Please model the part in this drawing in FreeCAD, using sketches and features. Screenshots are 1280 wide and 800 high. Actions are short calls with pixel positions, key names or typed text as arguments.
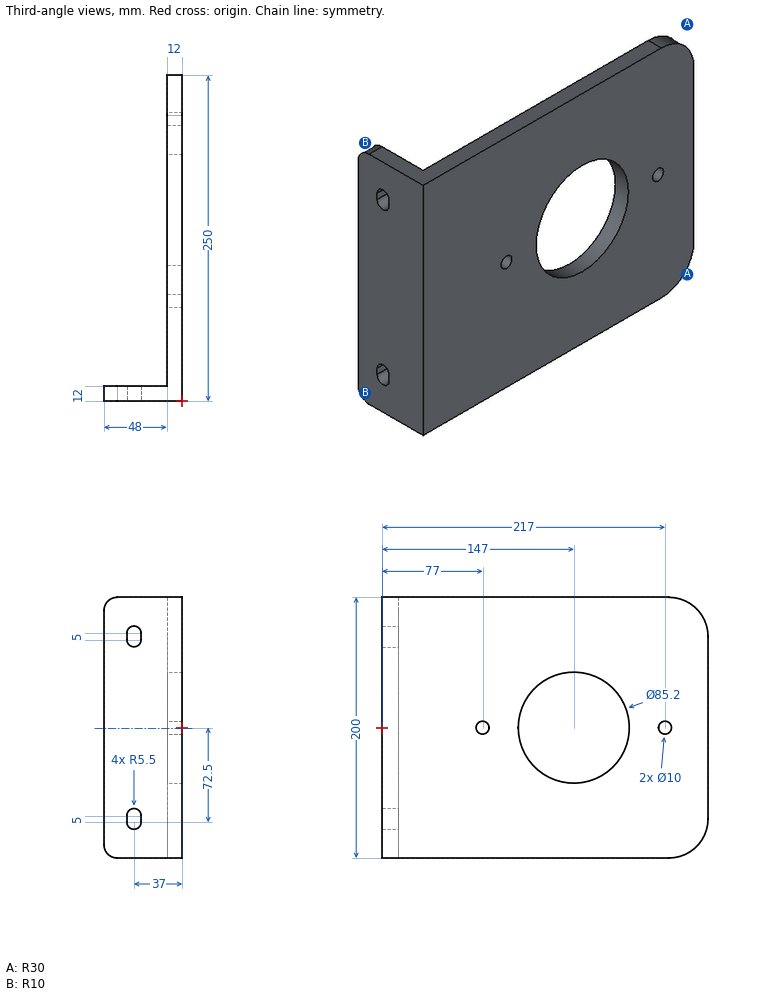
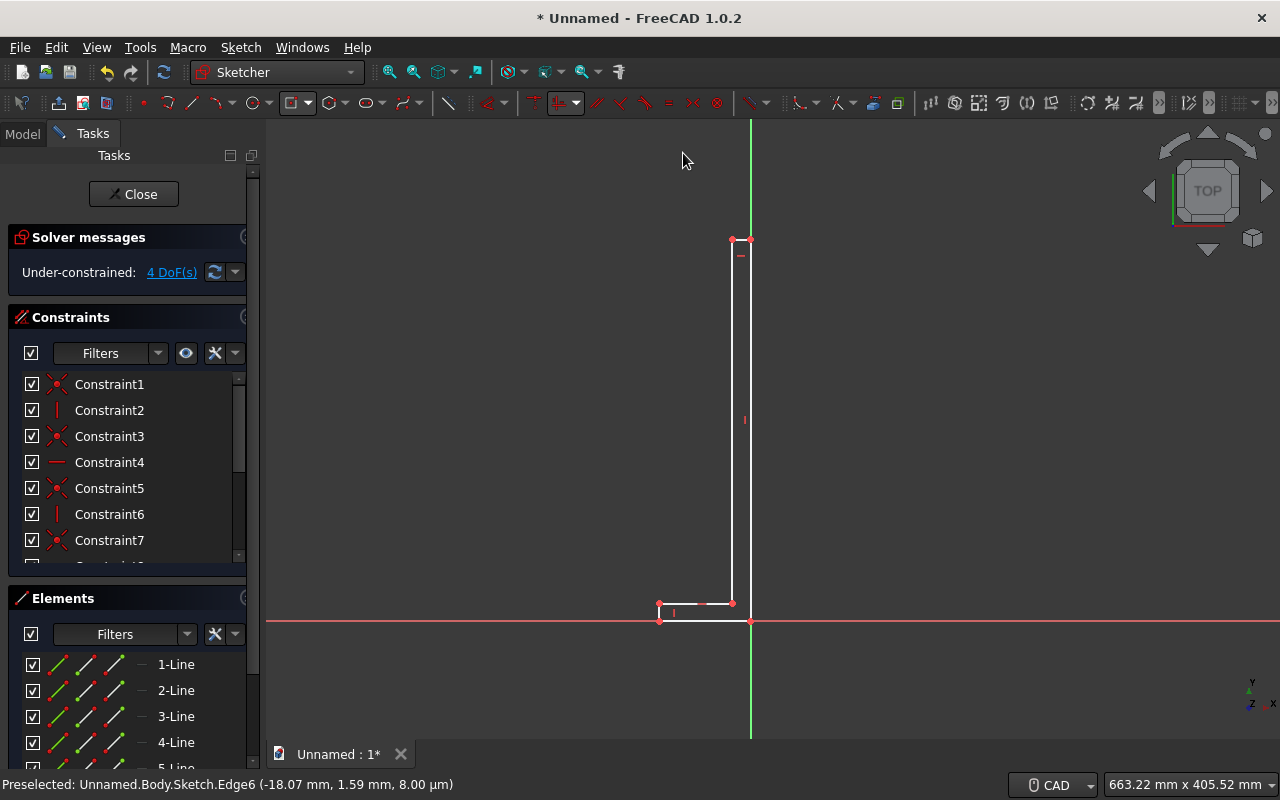
click(488, 104)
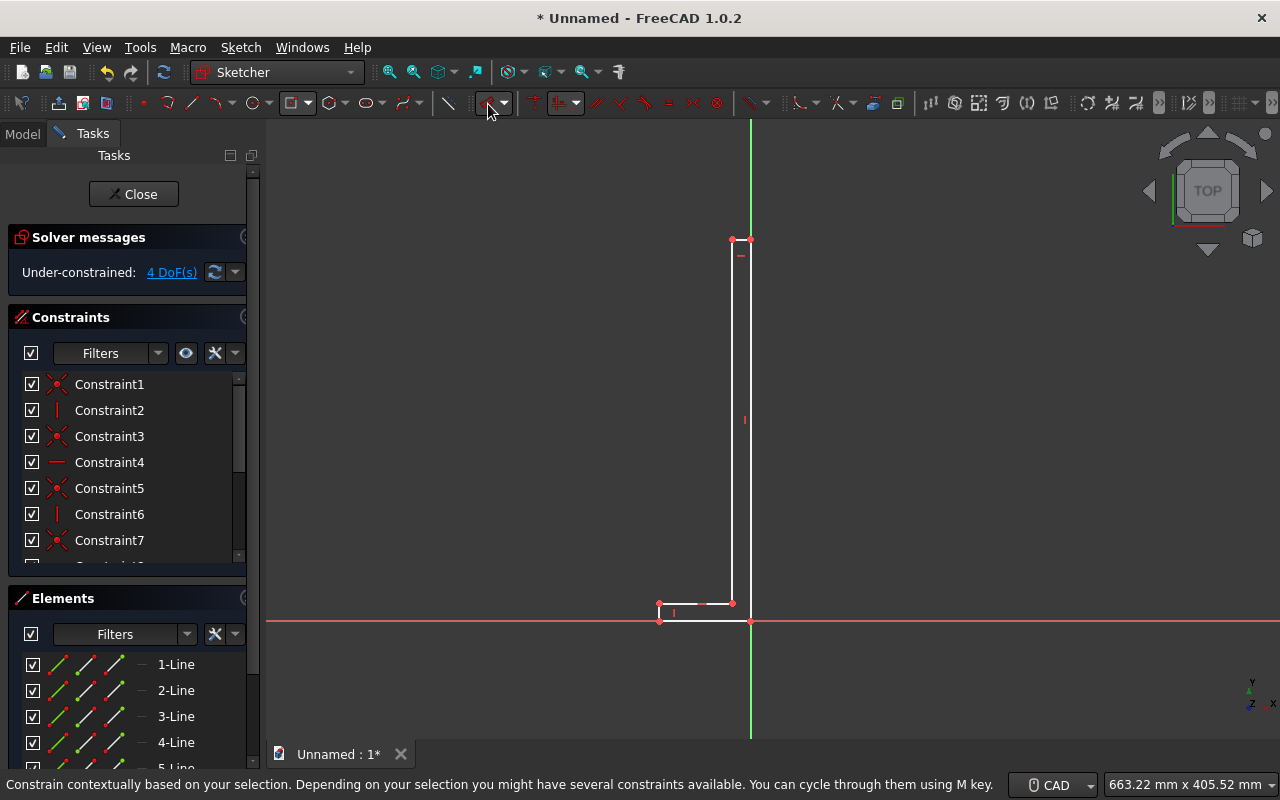
scroll(741, 240, up, 4)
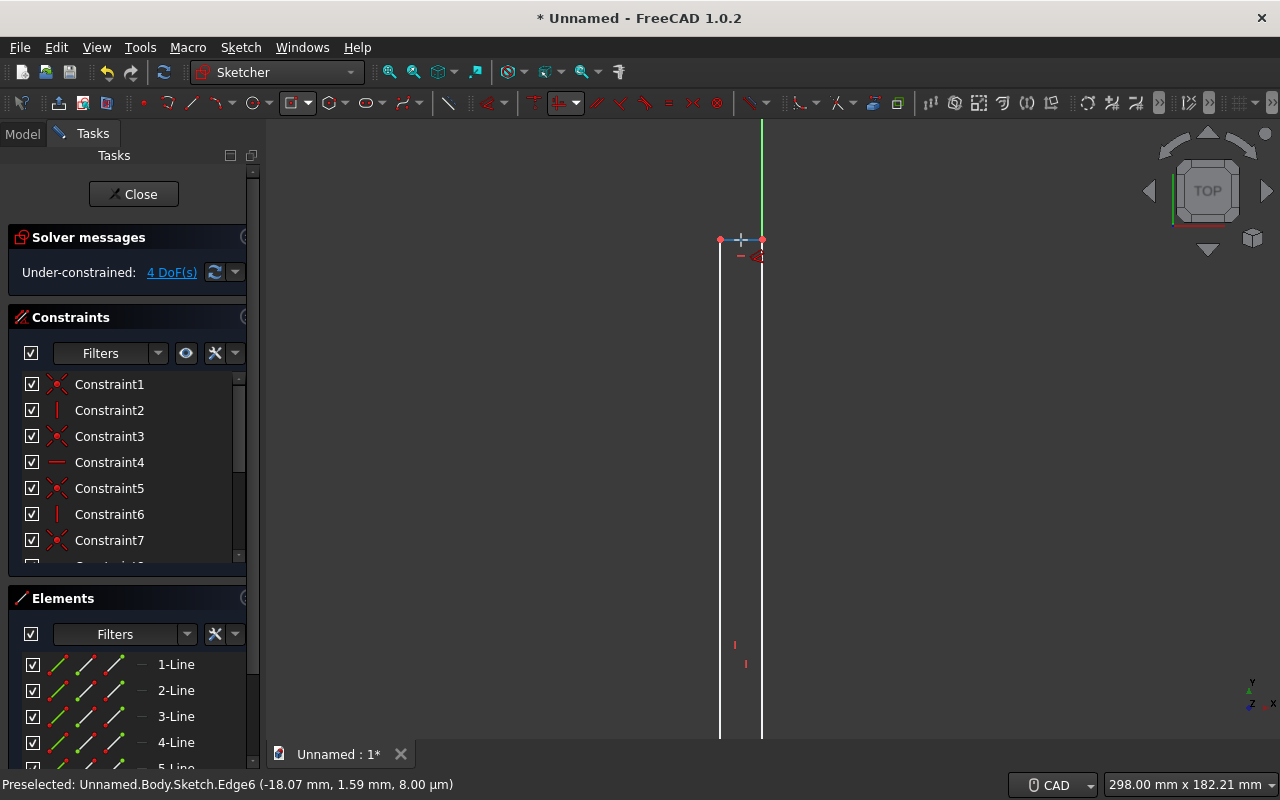
click(741, 240)
click(741, 206)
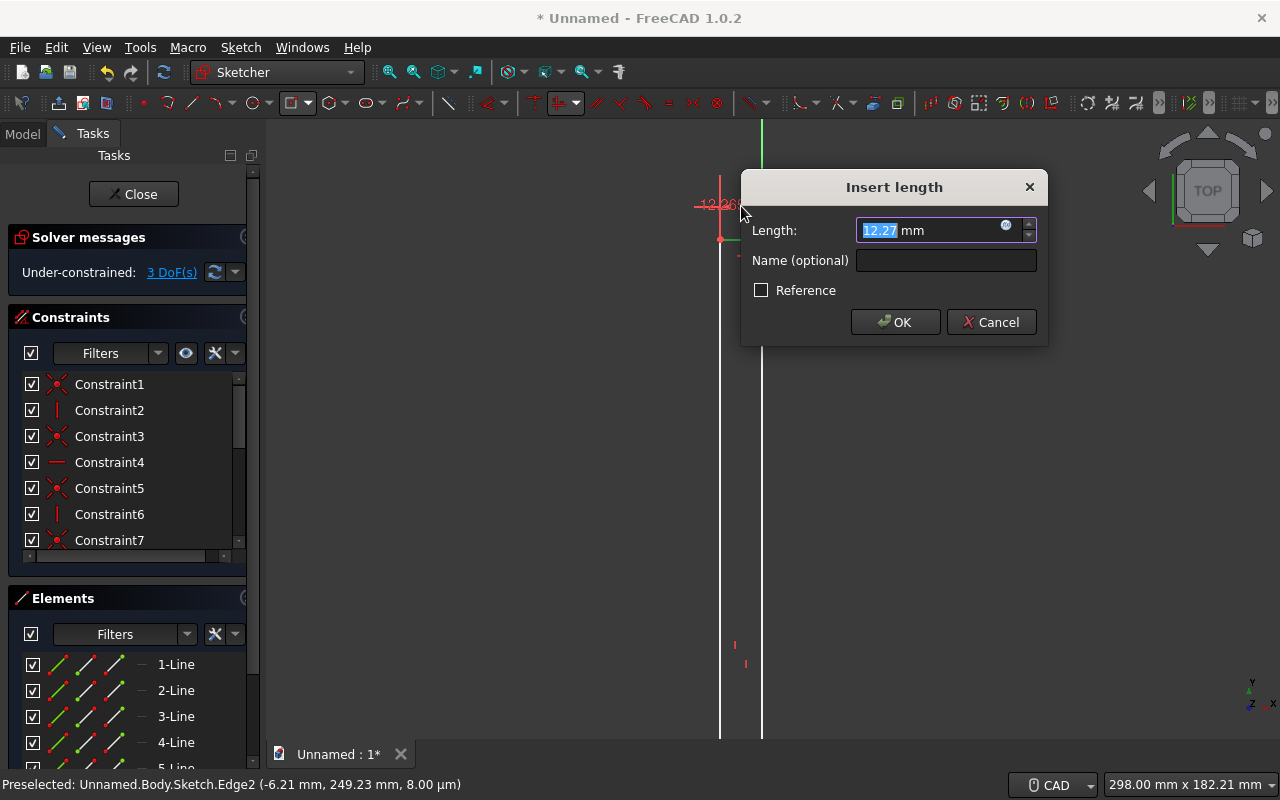
text(12)
key(Return)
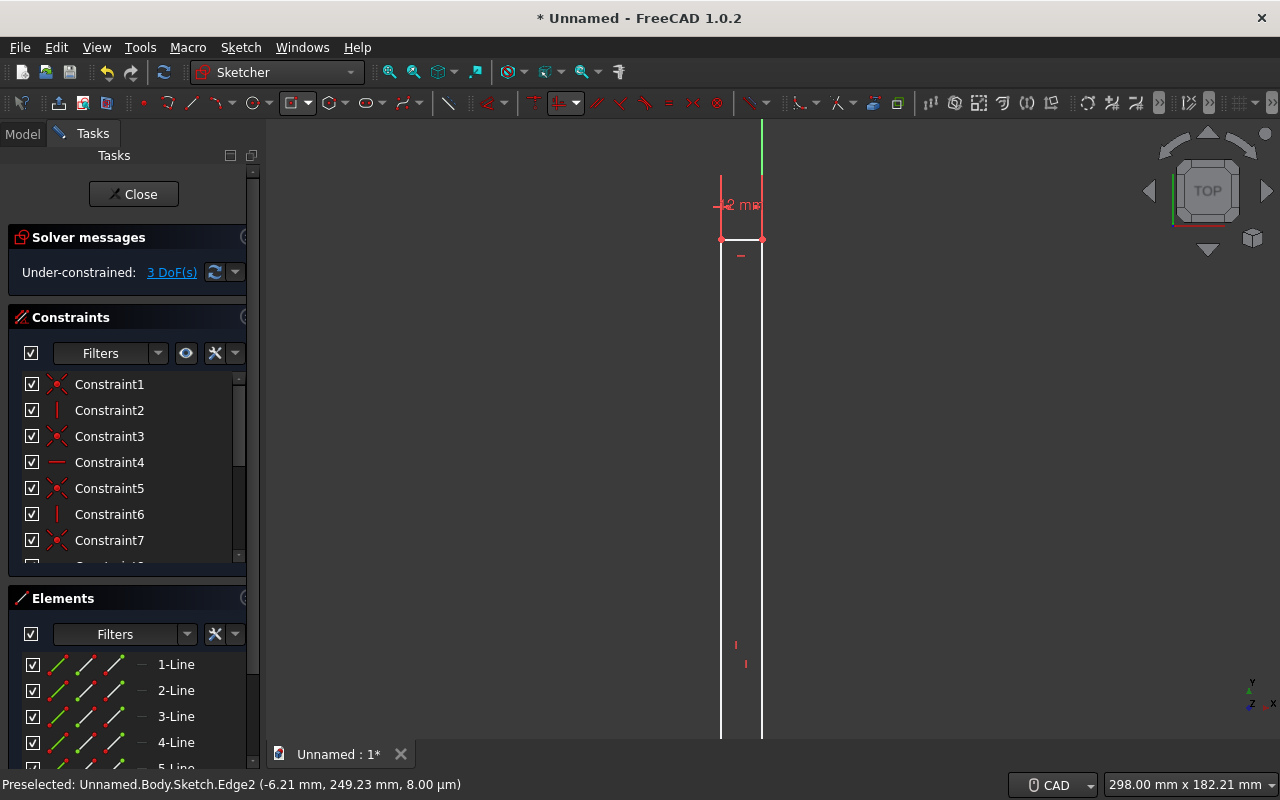
scroll(741, 238, down, 4)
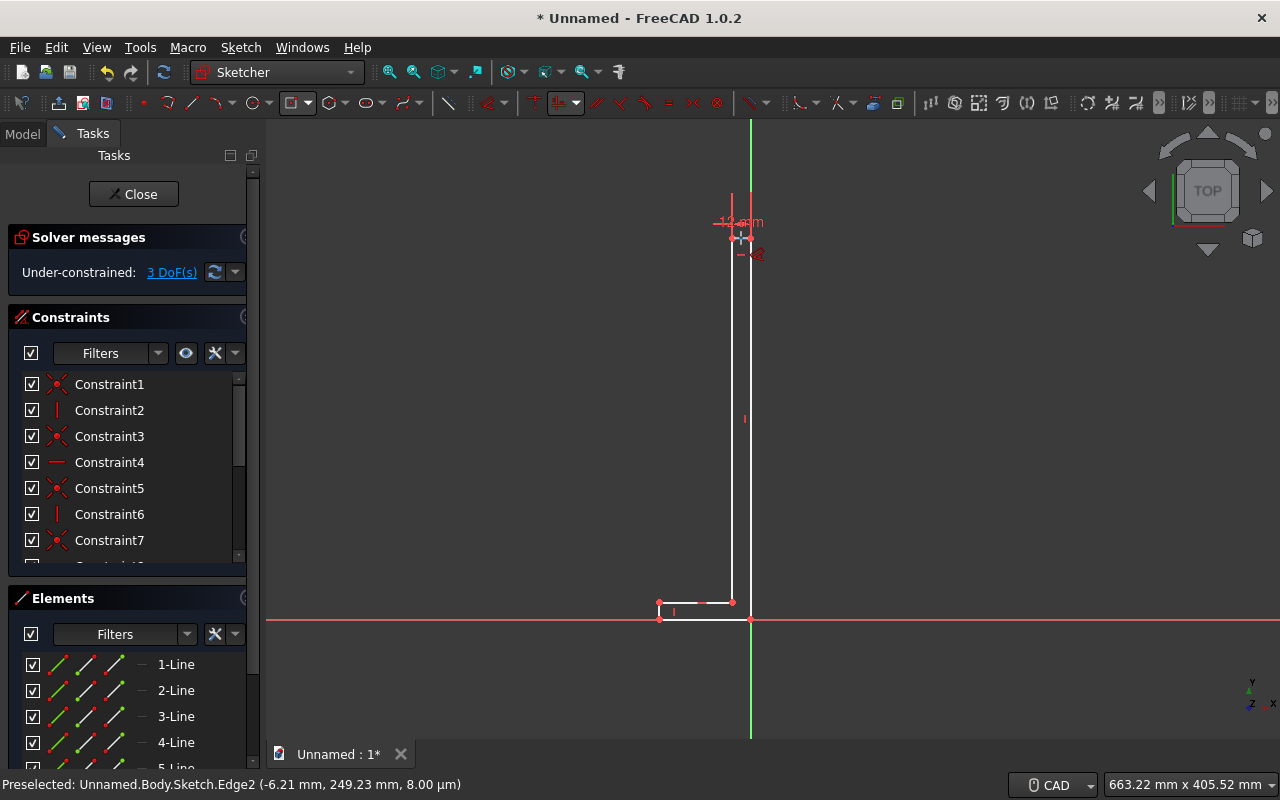
click(710, 603)
click(696, 637)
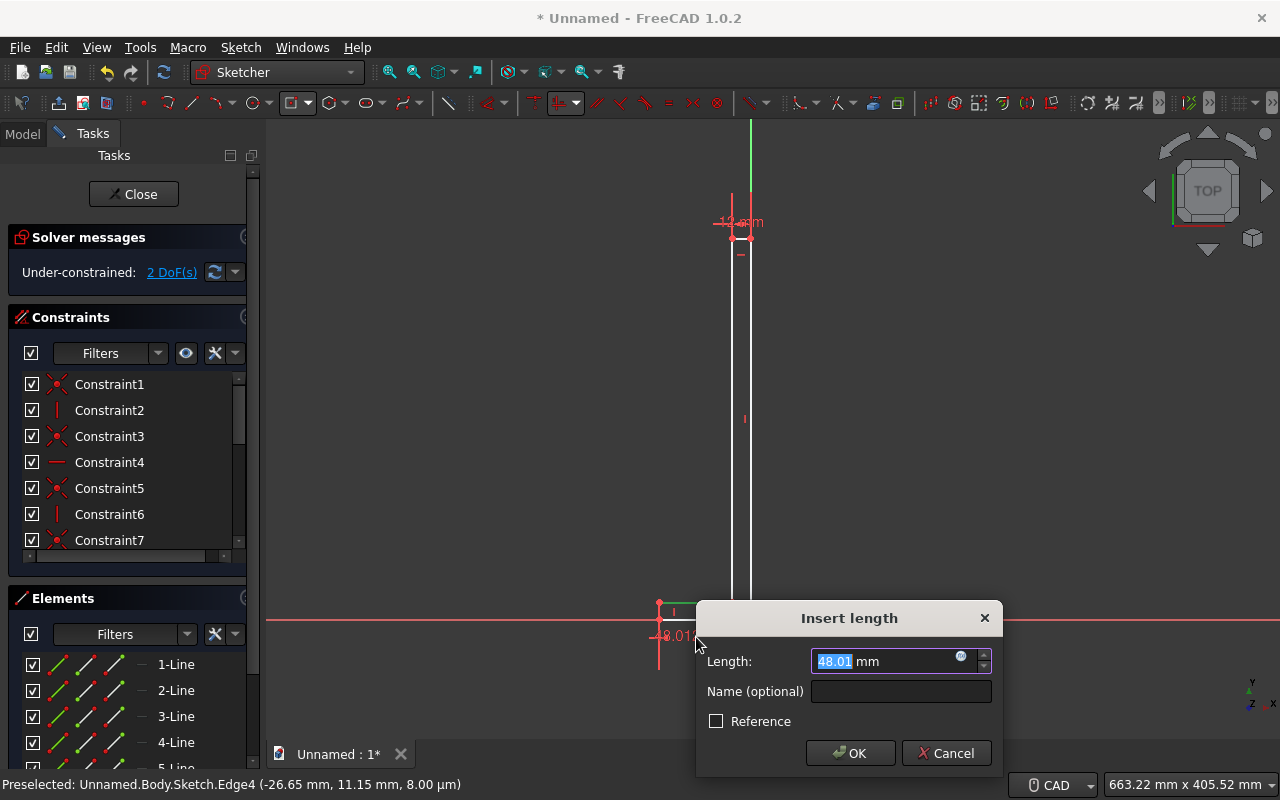
text(48)
key(Return)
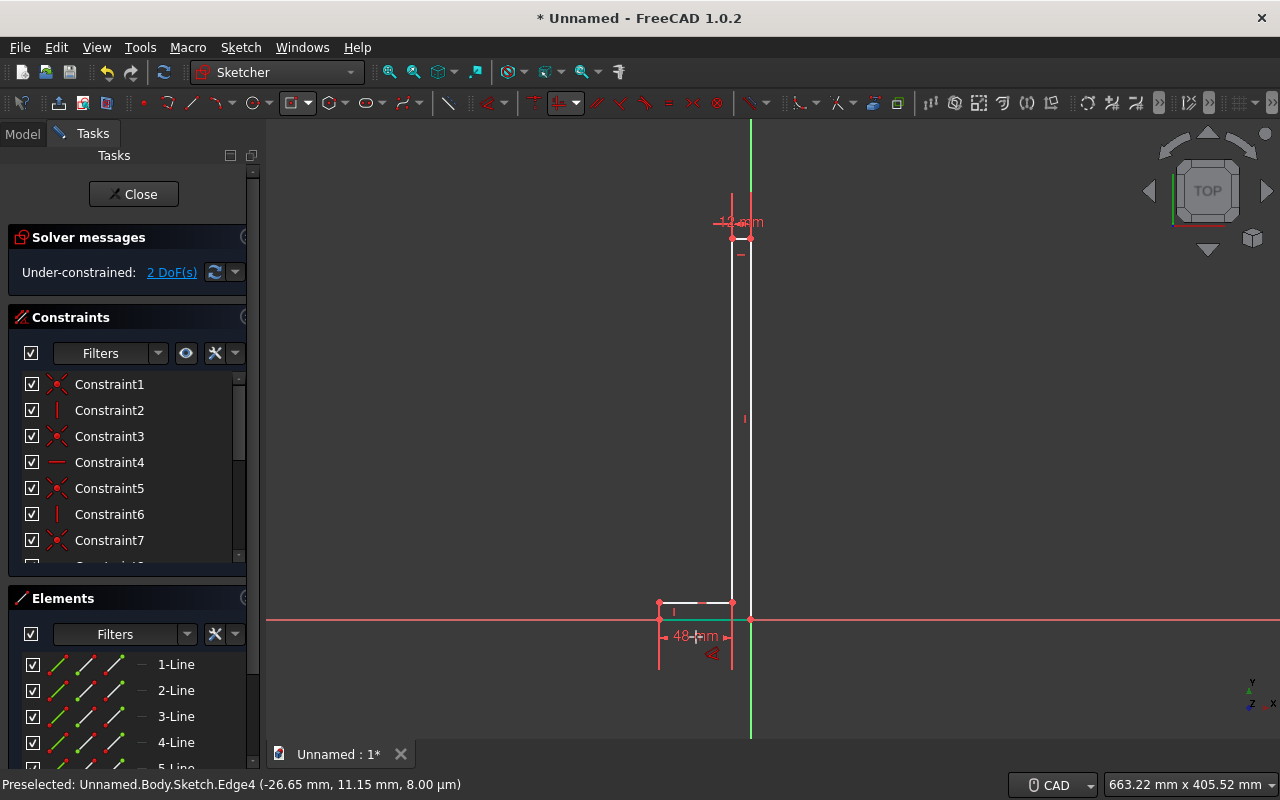
scroll(659, 611, up, 4)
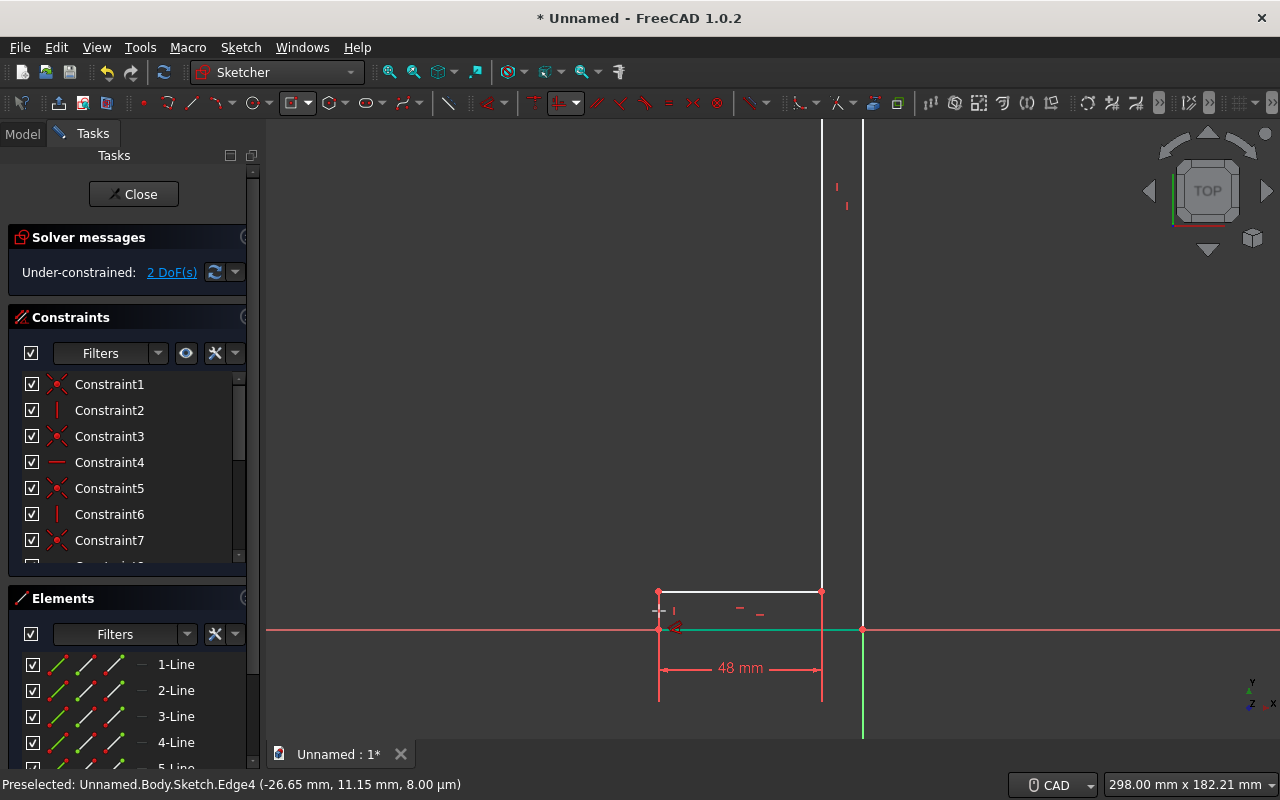
click(659, 611)
click(625, 611)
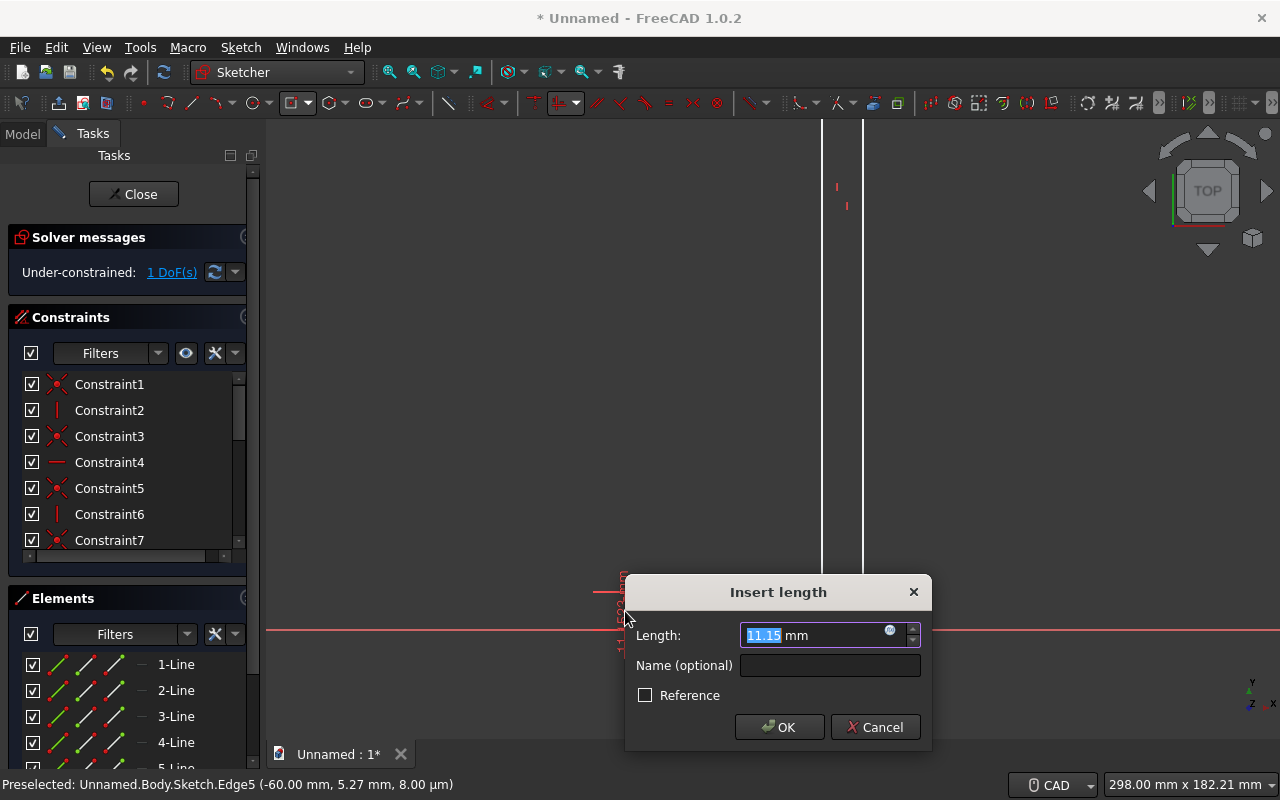
text(12)
key(Return)